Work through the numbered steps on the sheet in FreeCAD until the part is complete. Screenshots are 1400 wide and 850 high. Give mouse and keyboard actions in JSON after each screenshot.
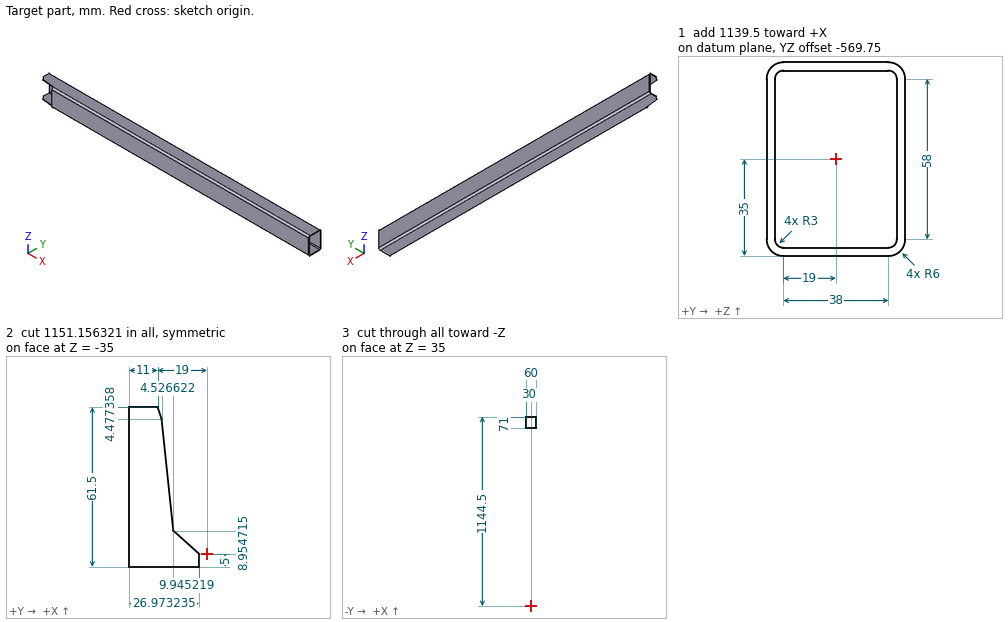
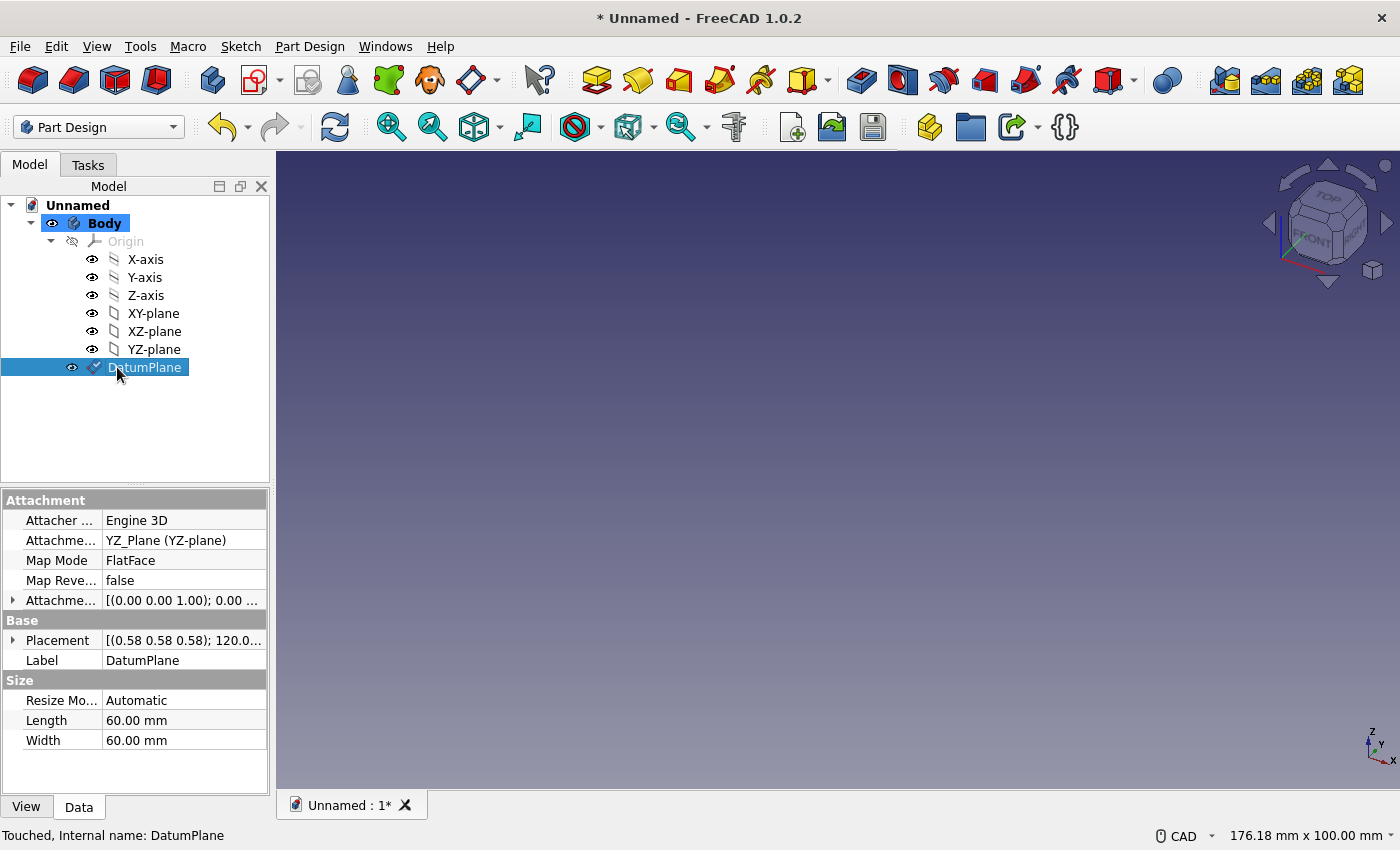
{"action": "left_click", "coordinate": [254, 80]}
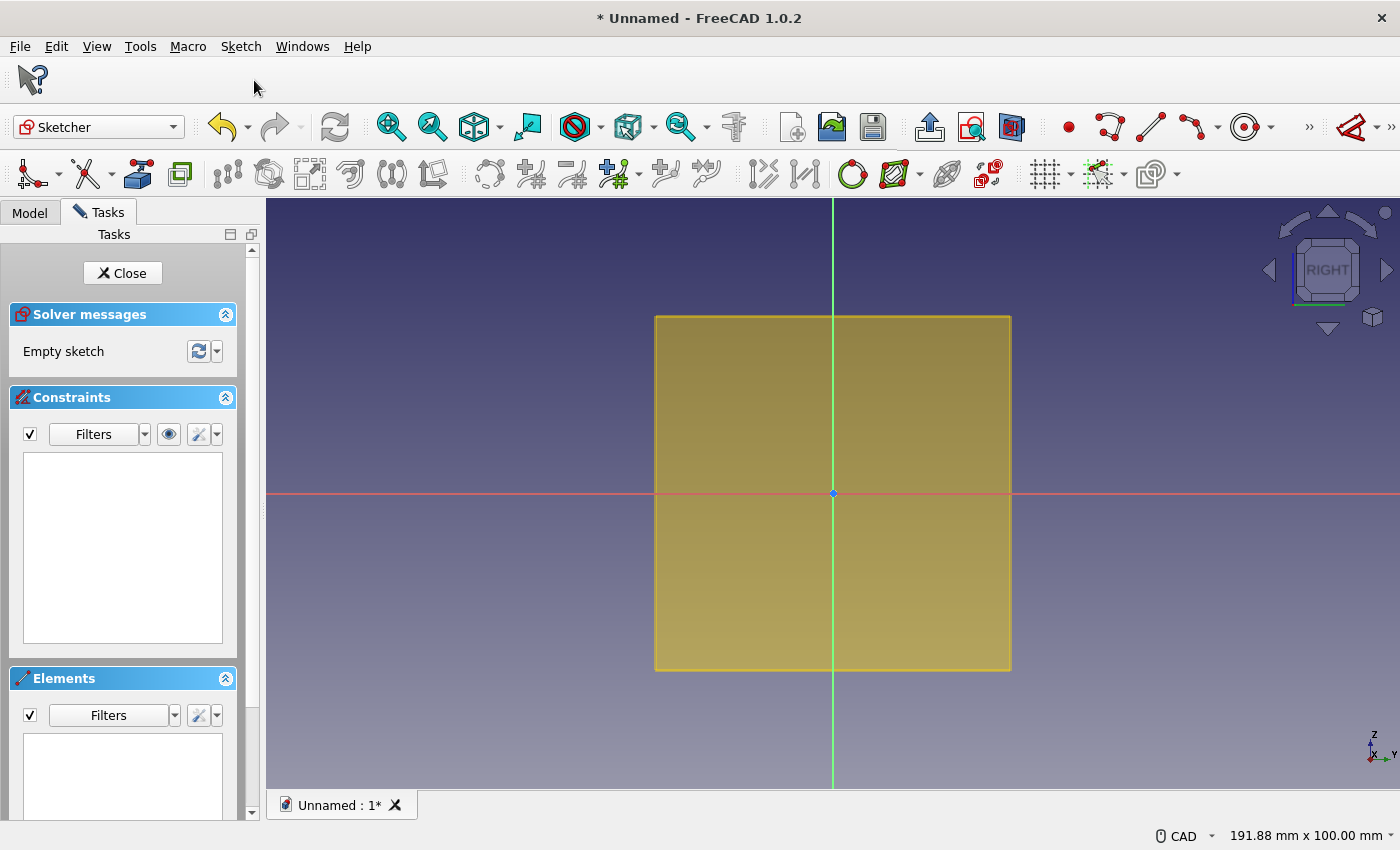
{"action": "key", "text": "g l"}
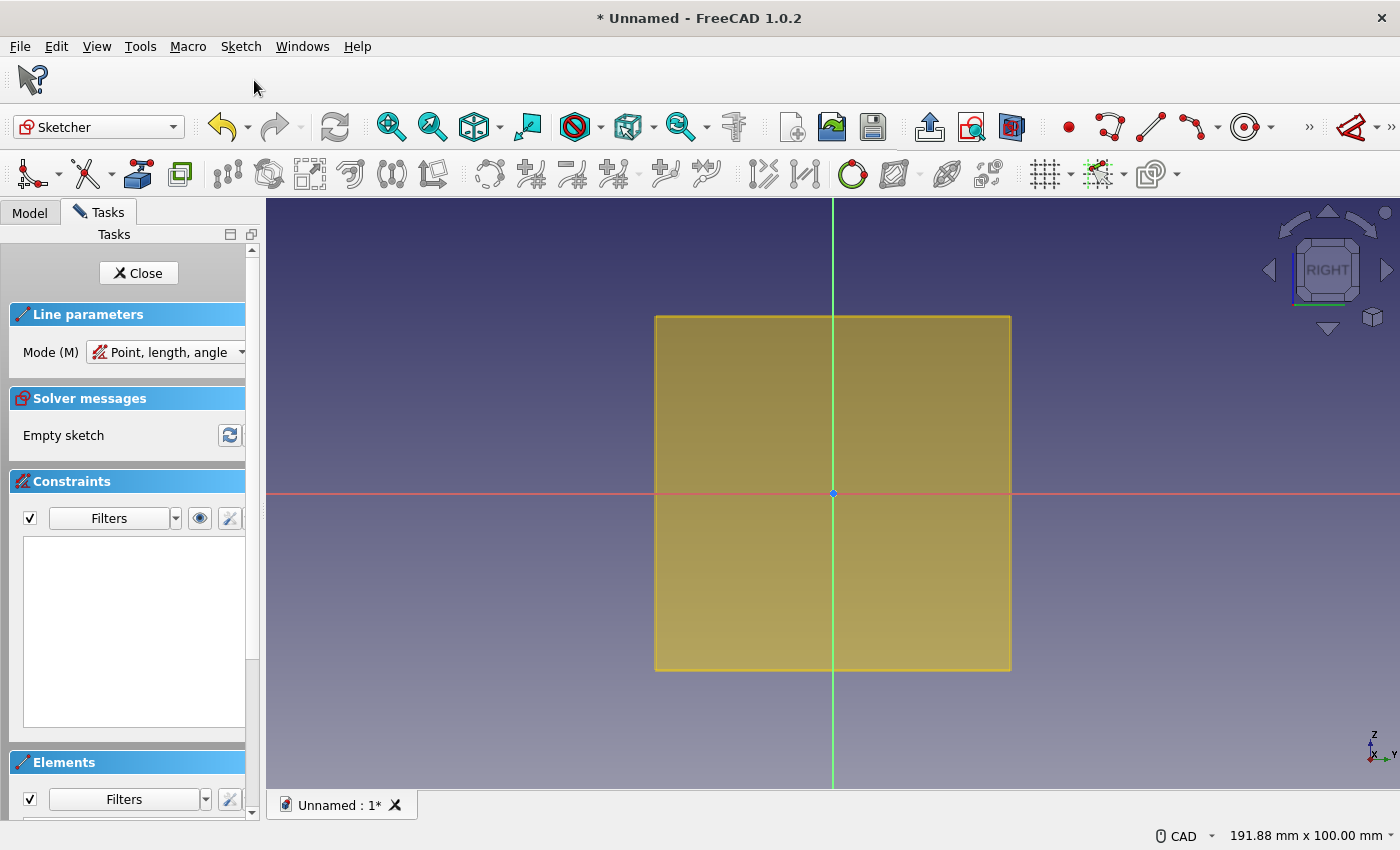
{"action": "left_click", "coordinate": [721, 700]}
{"action": "left_click", "coordinate": [945, 700]}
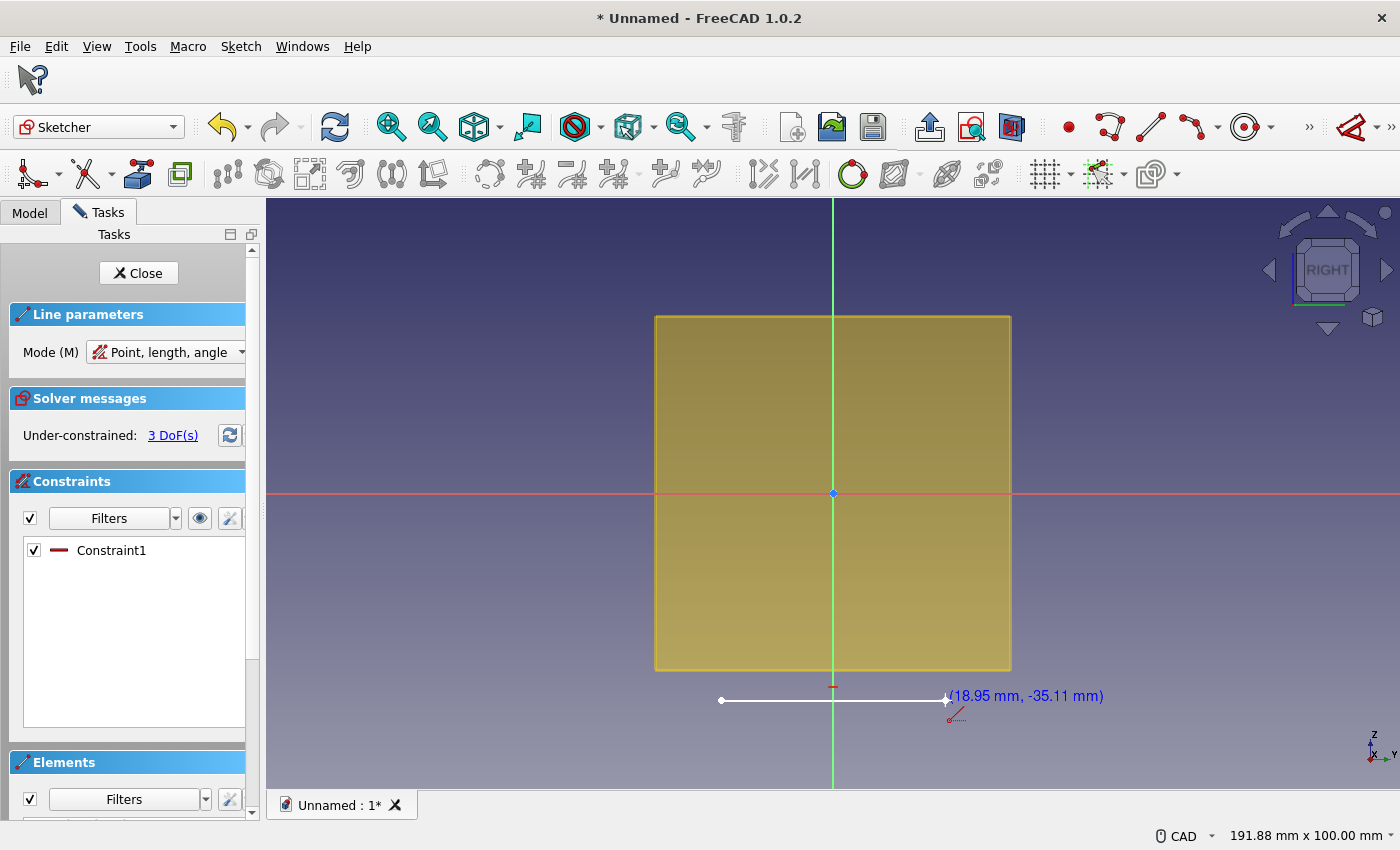
{"action": "left_click", "coordinate": [981, 665]}
{"action": "left_click", "coordinate": [981, 322]}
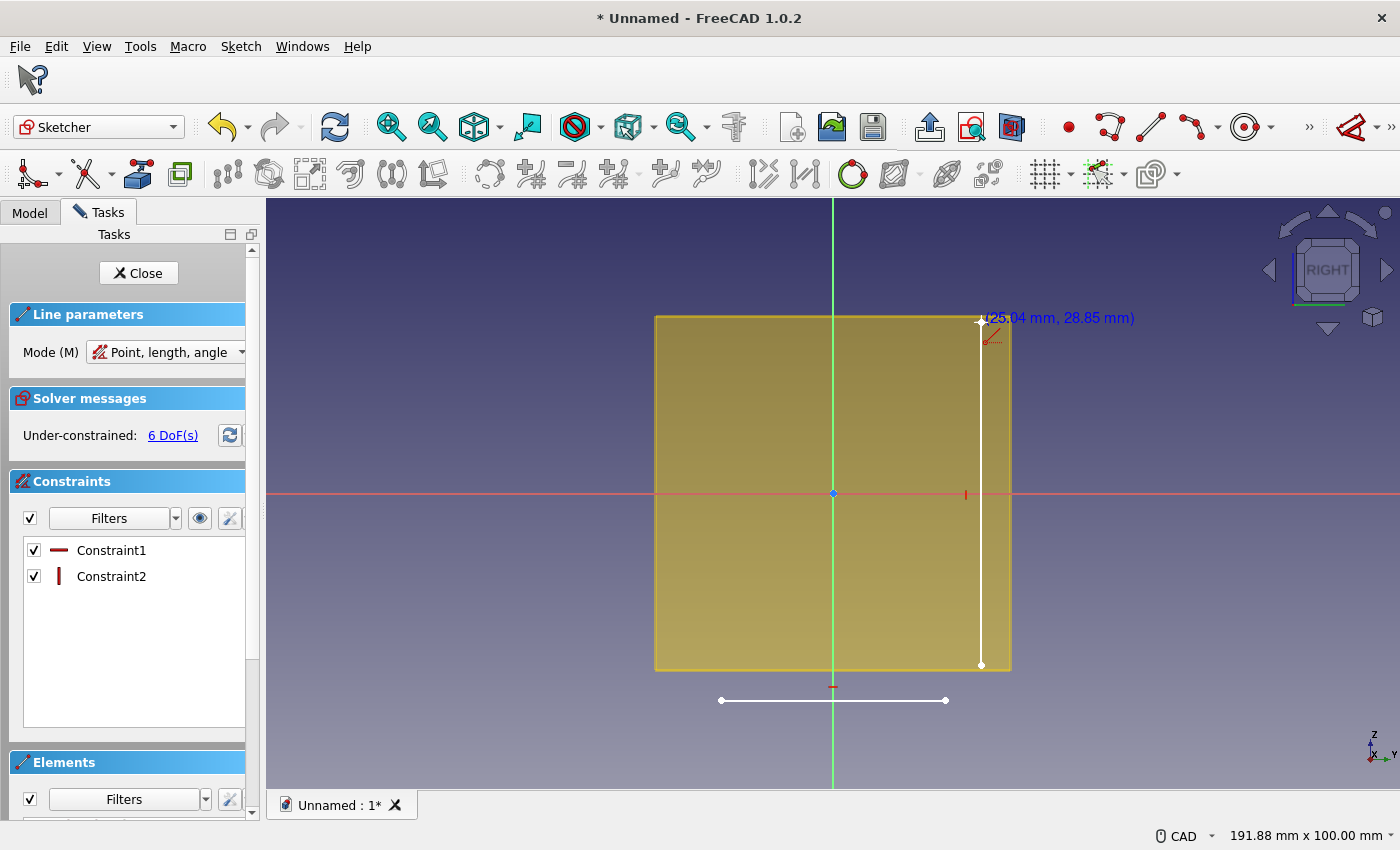
{"action": "left_click", "coordinate": [945, 287]}
{"action": "left_click", "coordinate": [721, 287]}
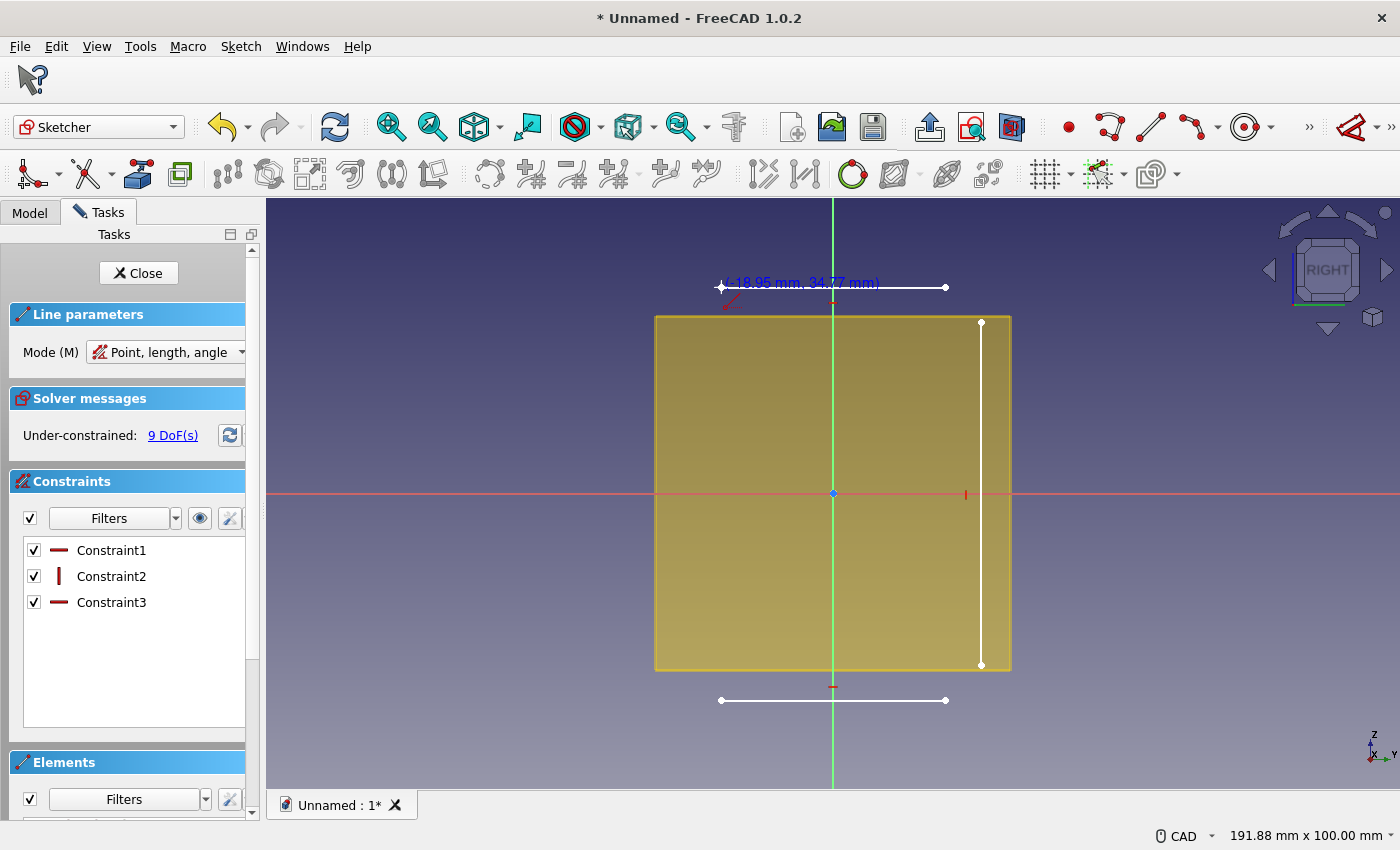
{"action": "left_click", "coordinate": [685, 322]}
{"action": "left_click", "coordinate": [685, 665]}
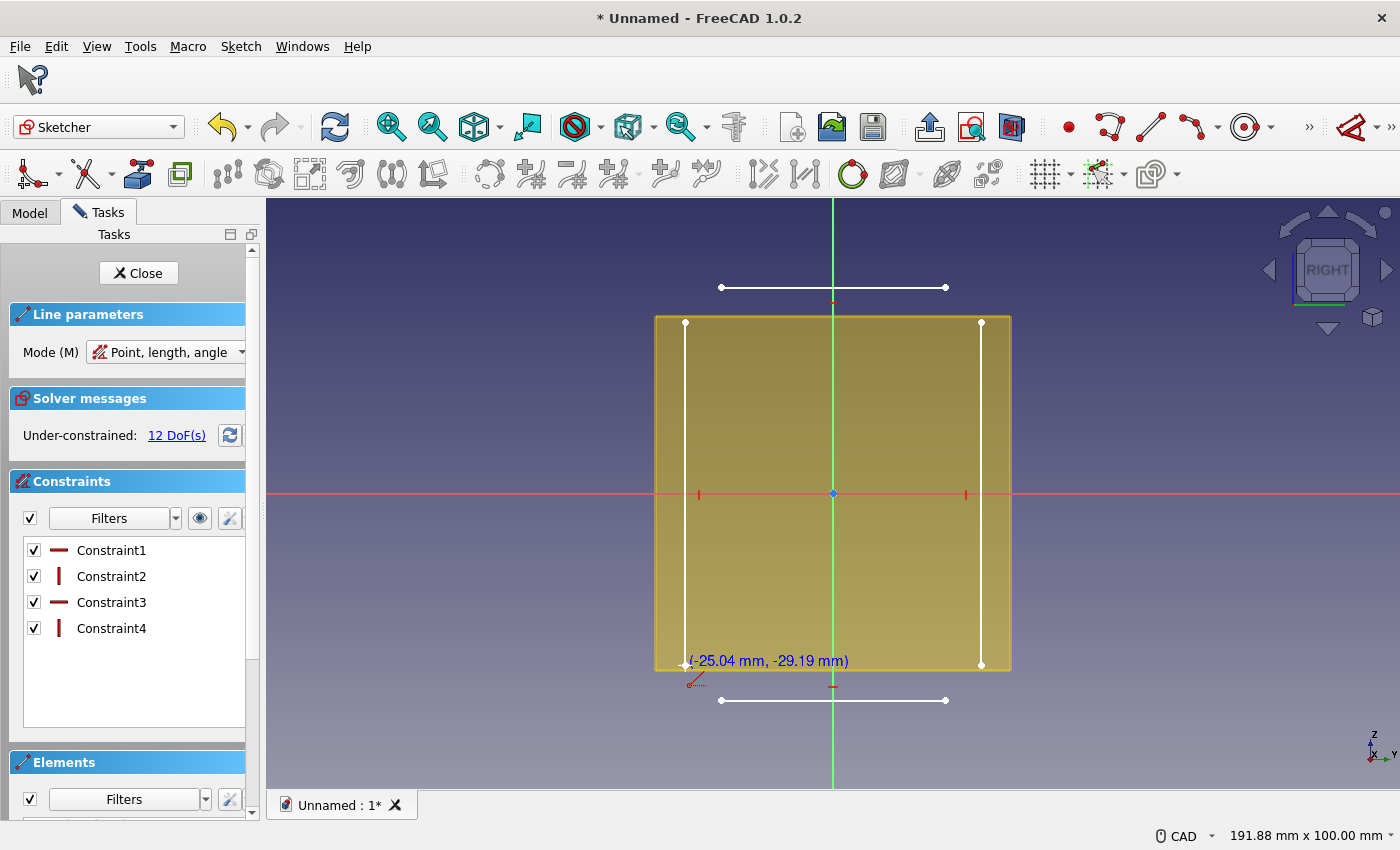
{"action": "key", "text": "g 3 a"}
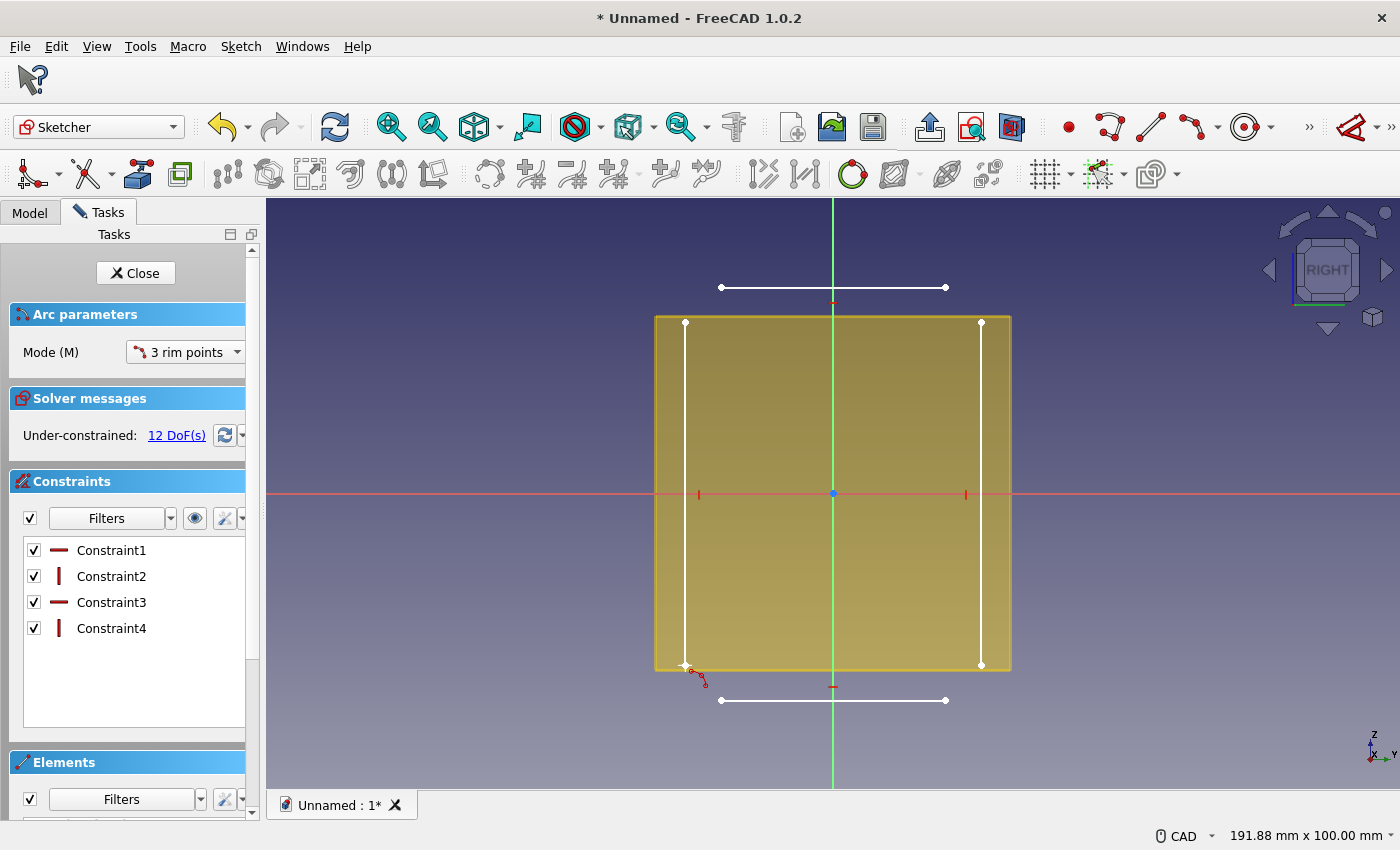
{"action": "left_click", "coordinate": [945, 701]}
{"action": "left_click", "coordinate": [981, 666]}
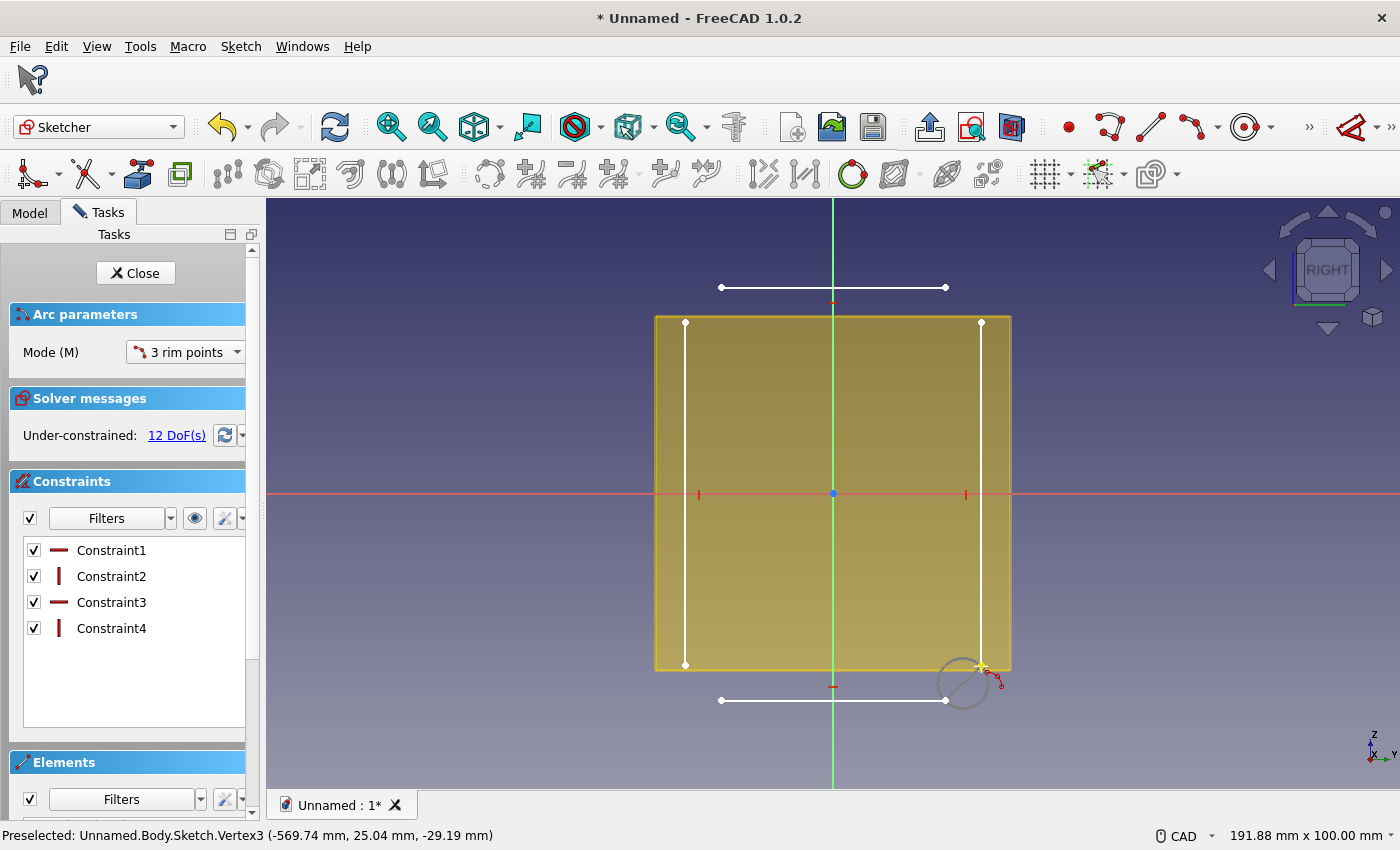
{"action": "scroll", "coordinate": [970, 690], "scroll_direction": "up", "scroll_amount": 3}